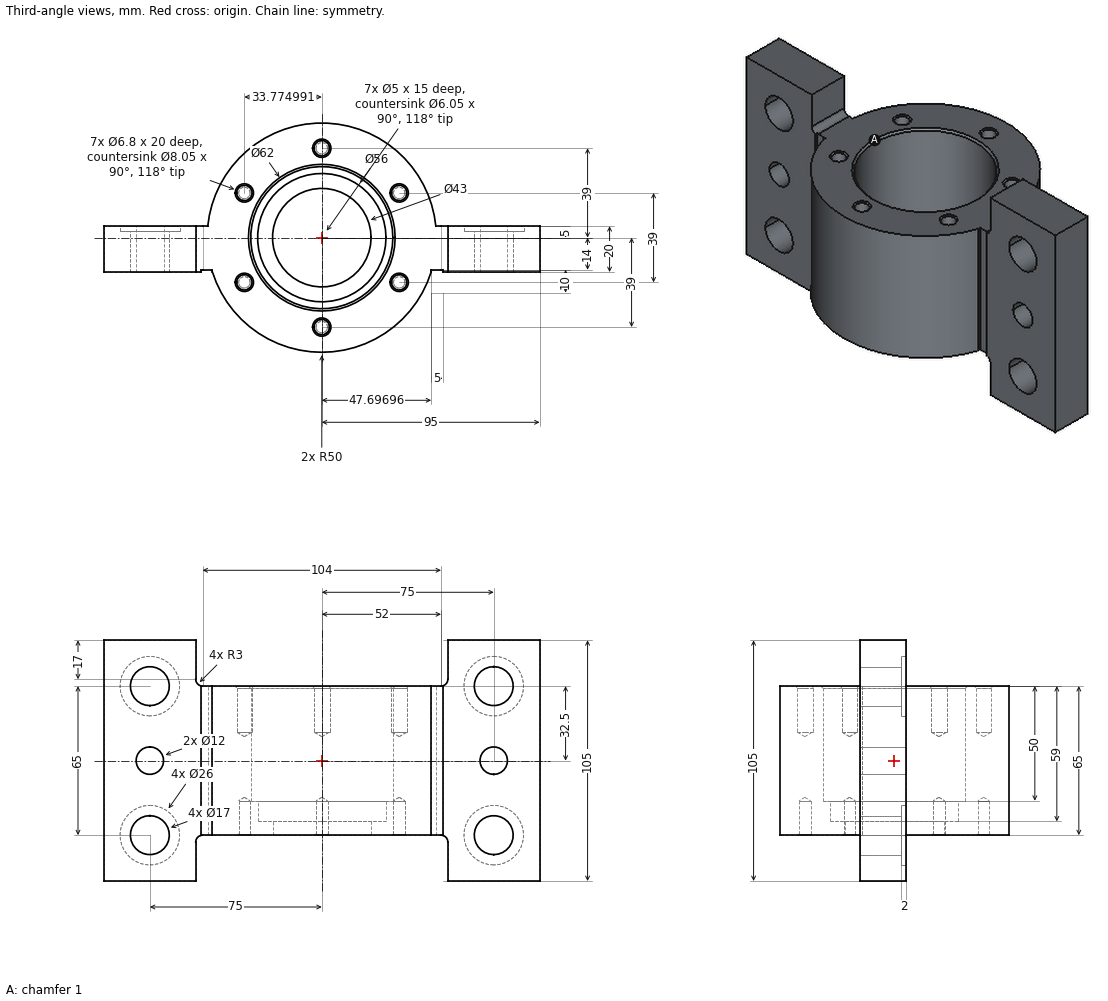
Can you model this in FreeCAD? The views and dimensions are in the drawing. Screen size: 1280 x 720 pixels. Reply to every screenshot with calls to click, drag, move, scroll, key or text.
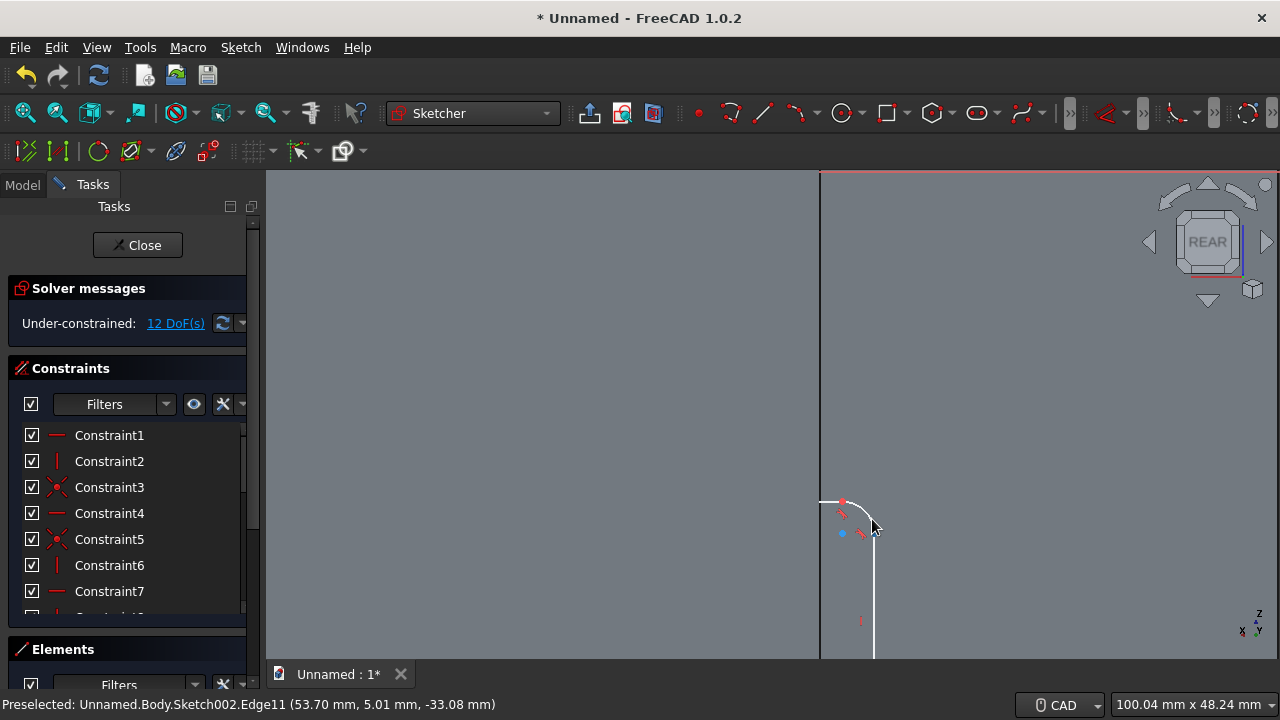
click(871, 519)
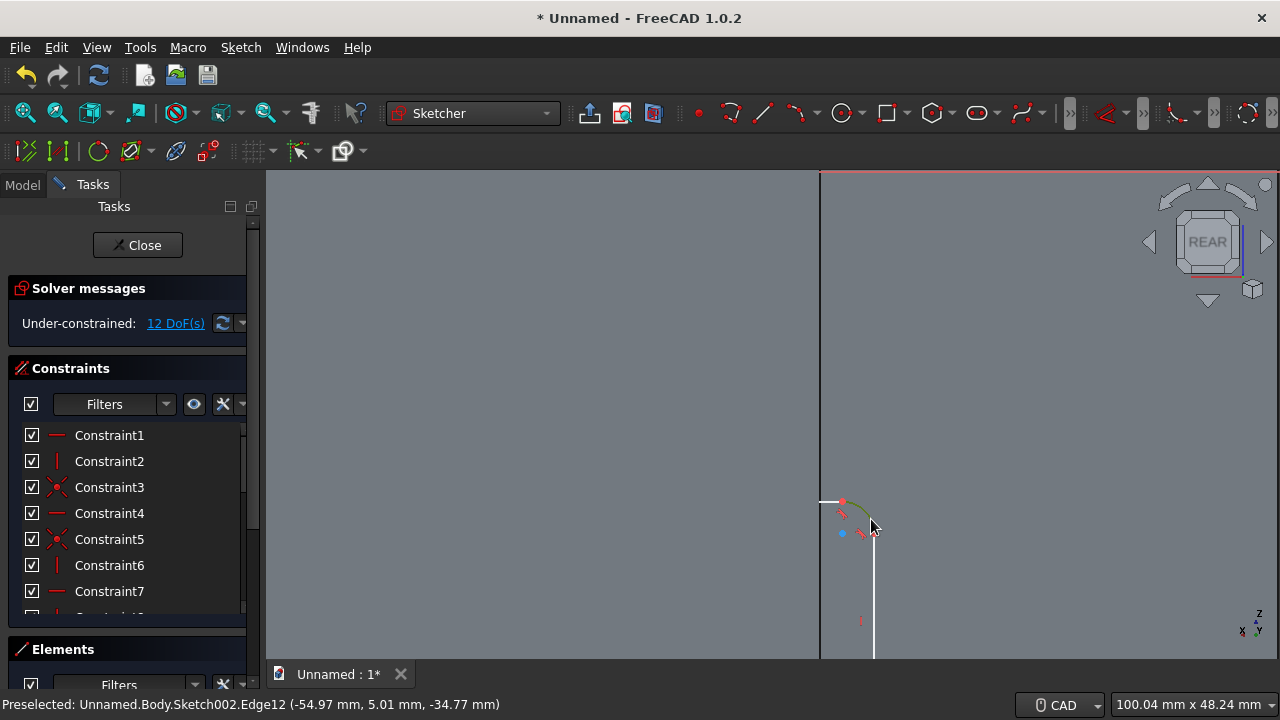
key(e)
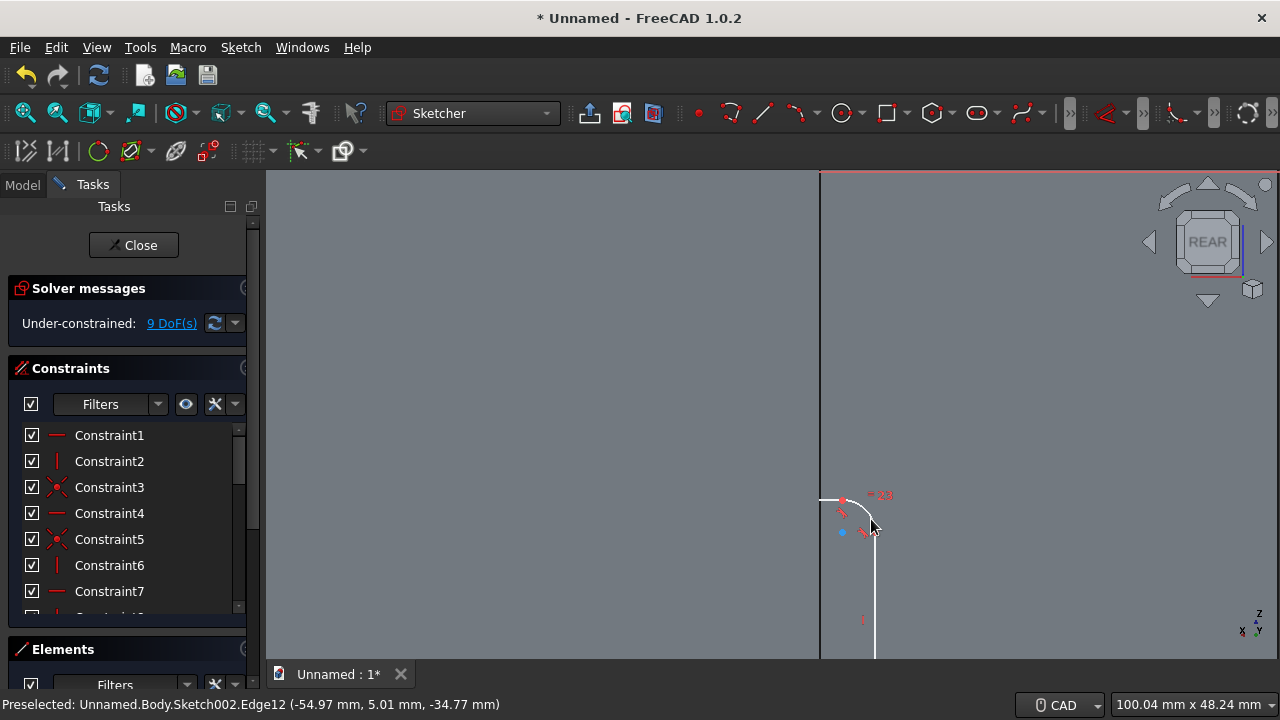
scroll(872, 519, down, 6)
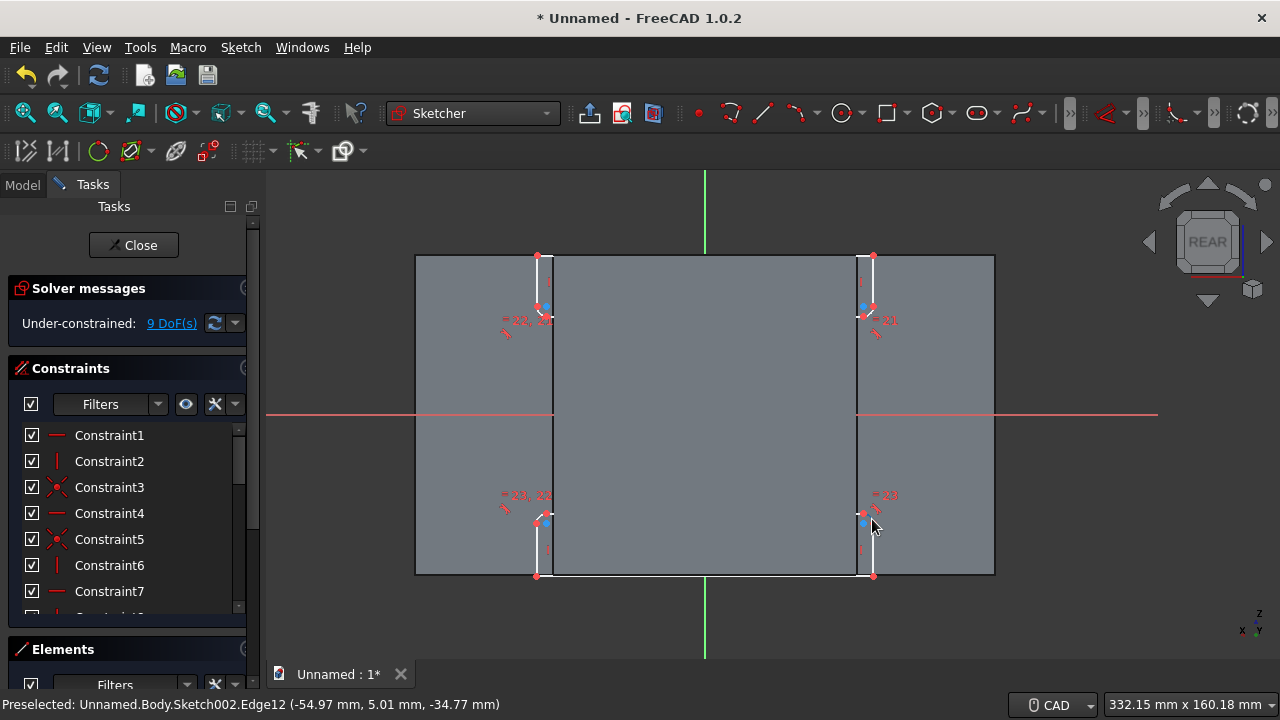
scroll(547, 307, up, 2)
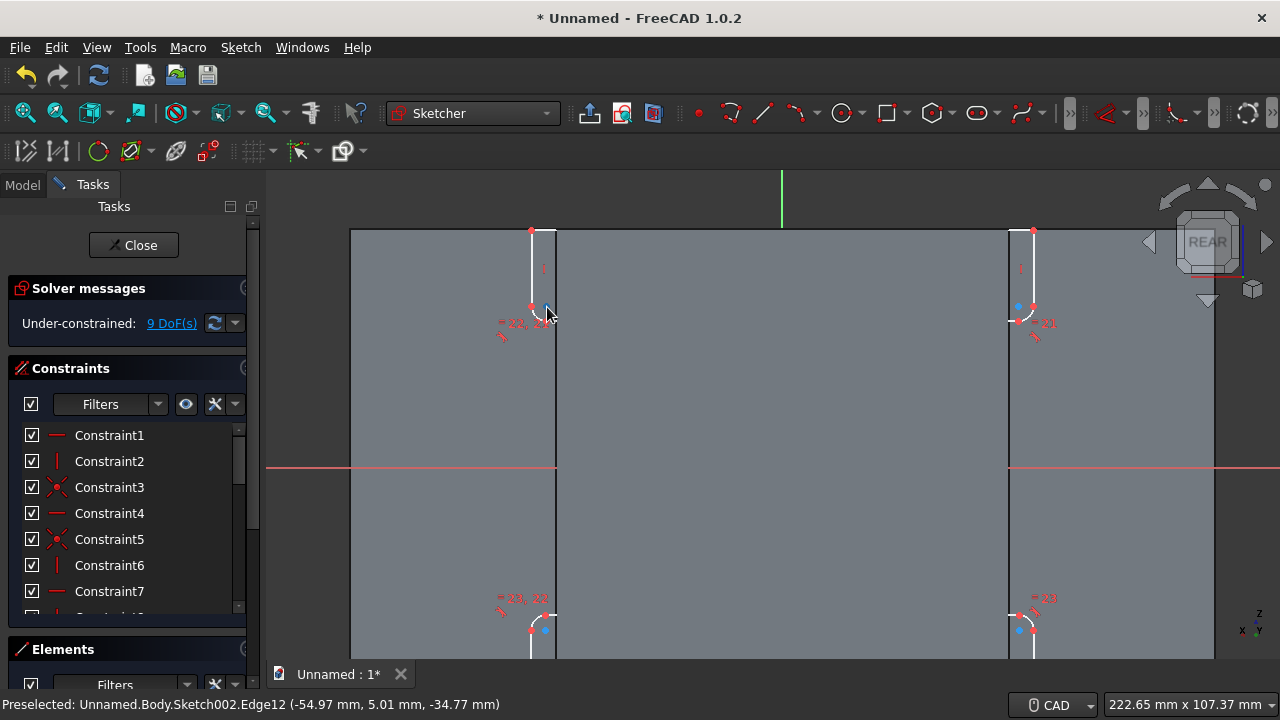
click(547, 306)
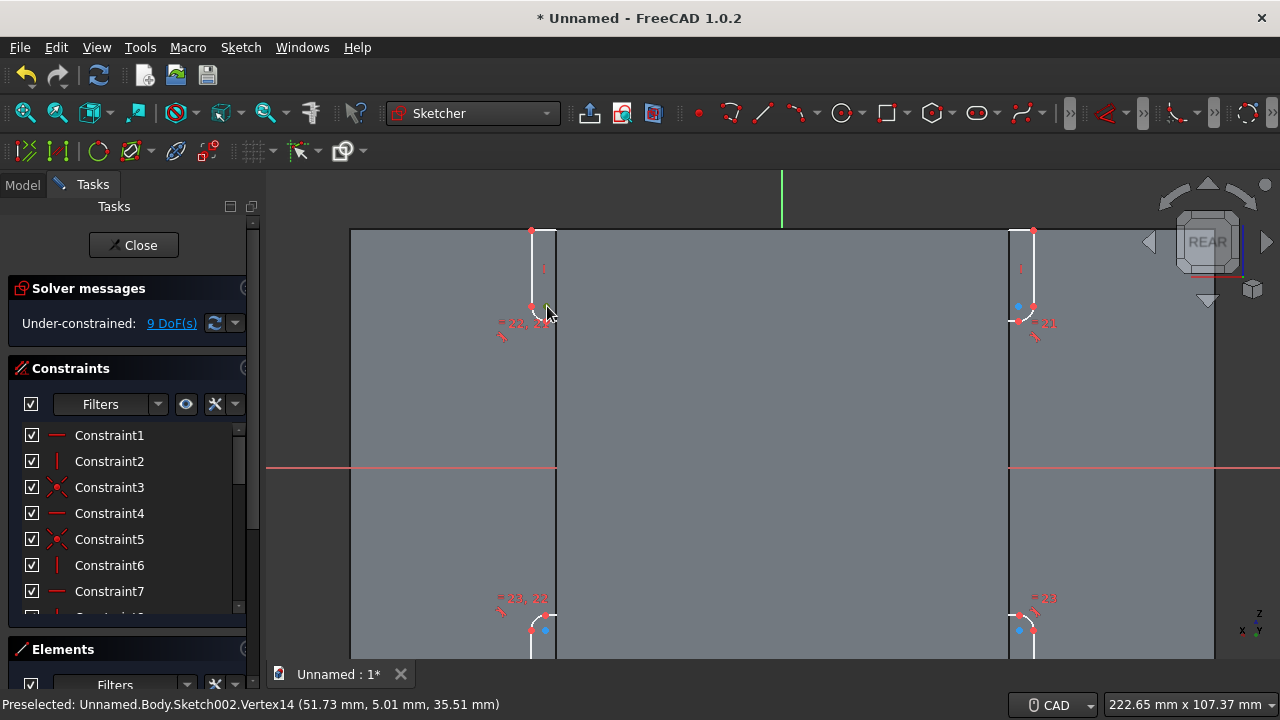
click(546, 630)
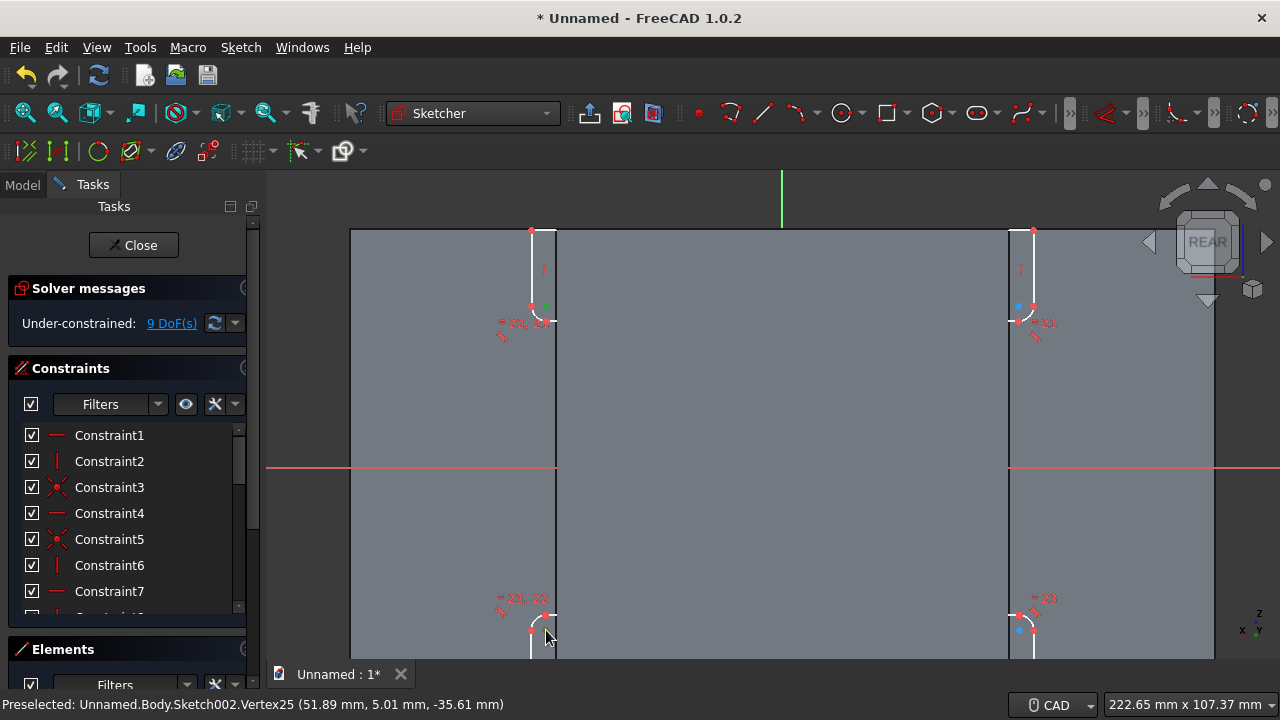
click(353, 468)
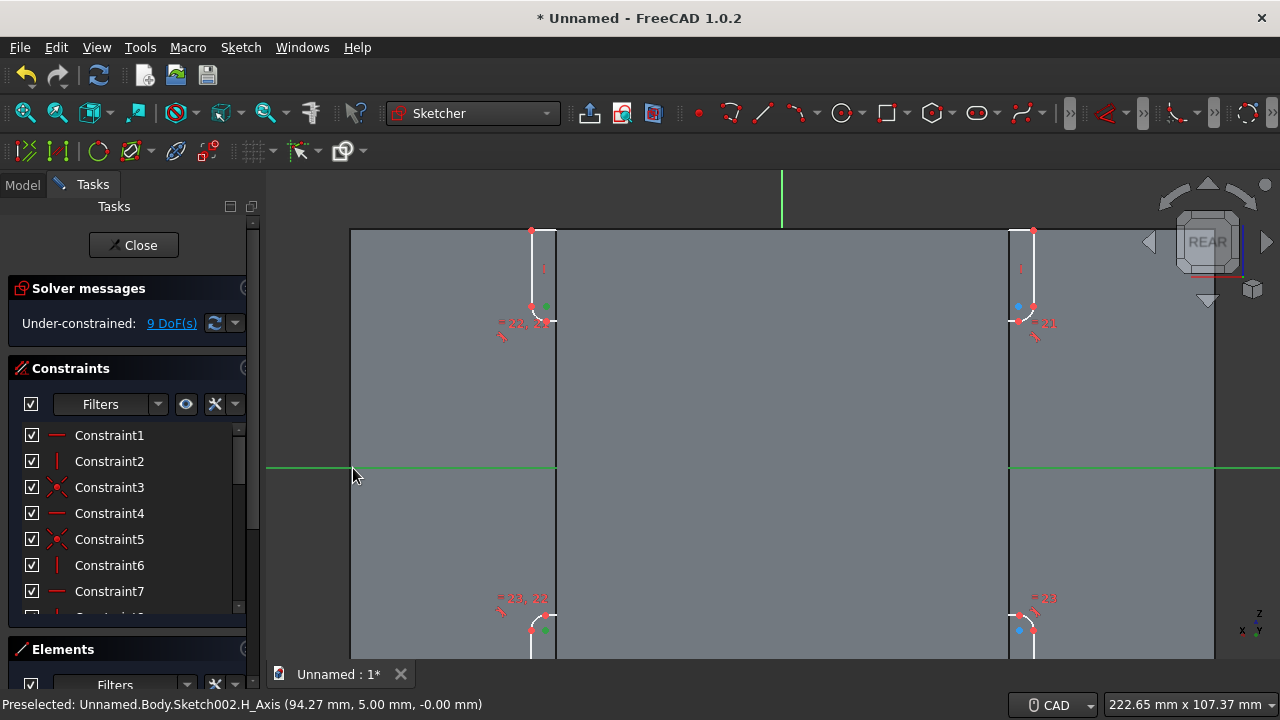
key(s)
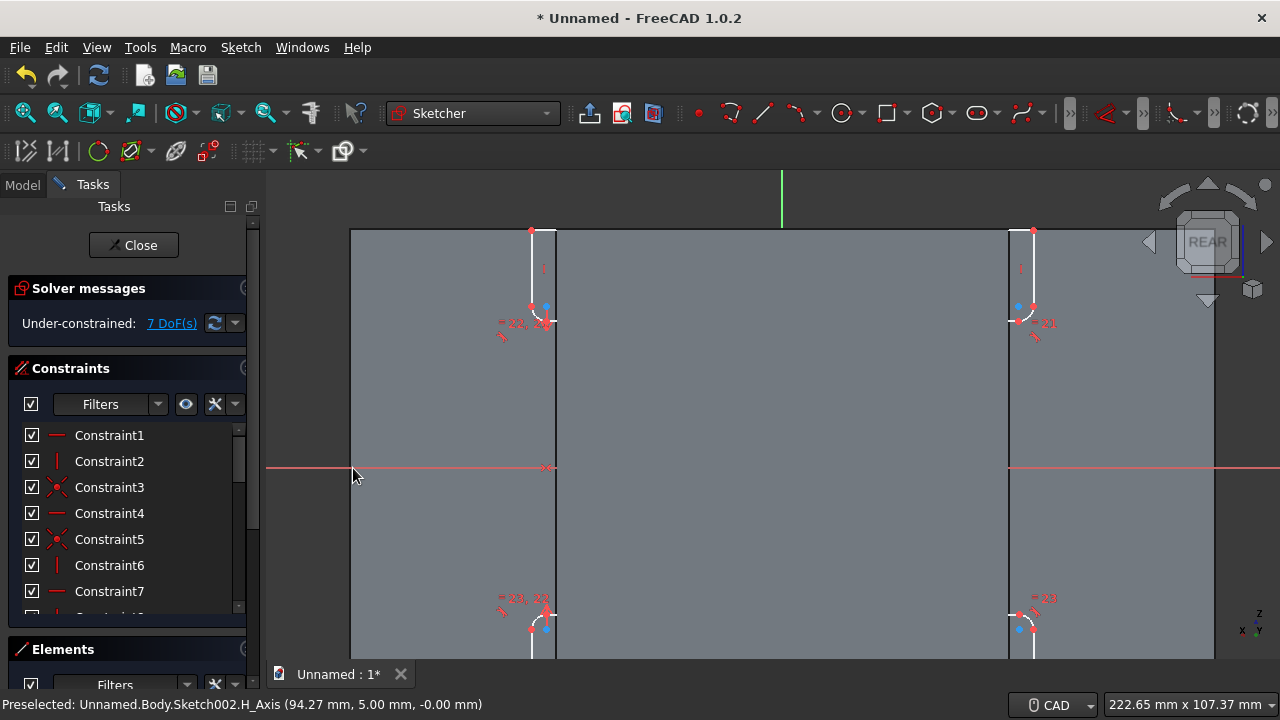
click(1034, 230)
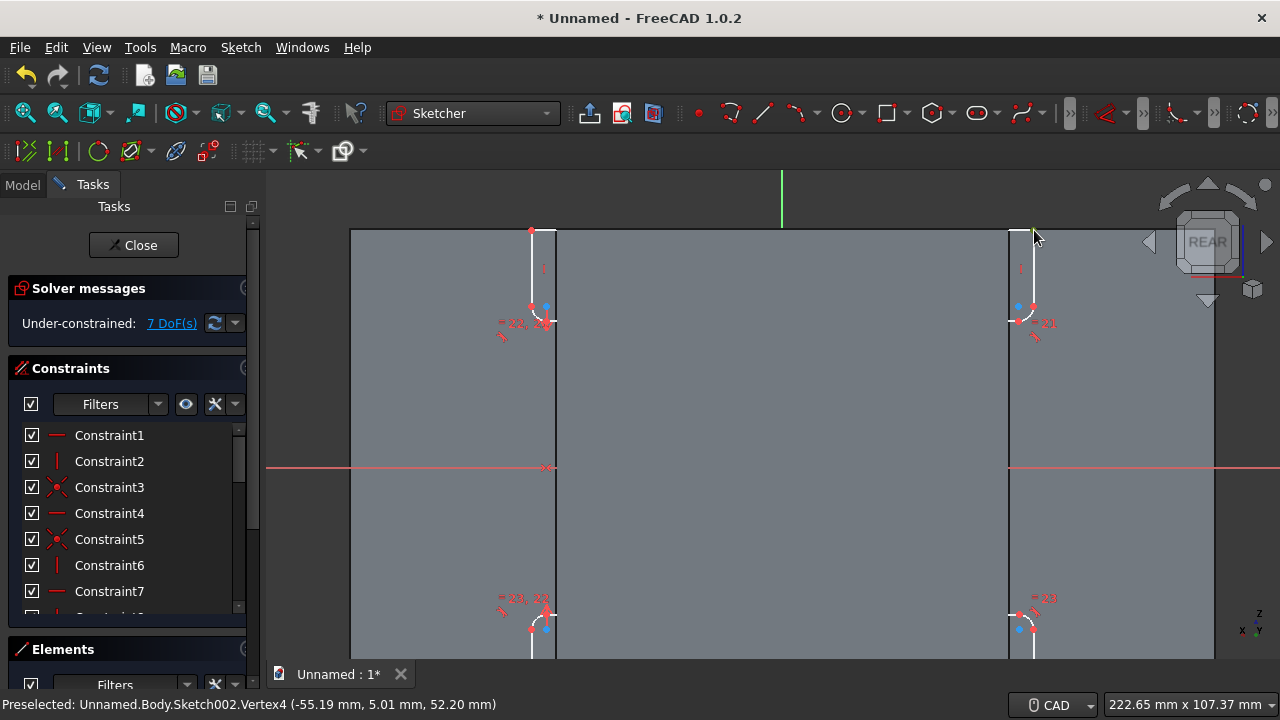
scroll(546, 306, down, 2)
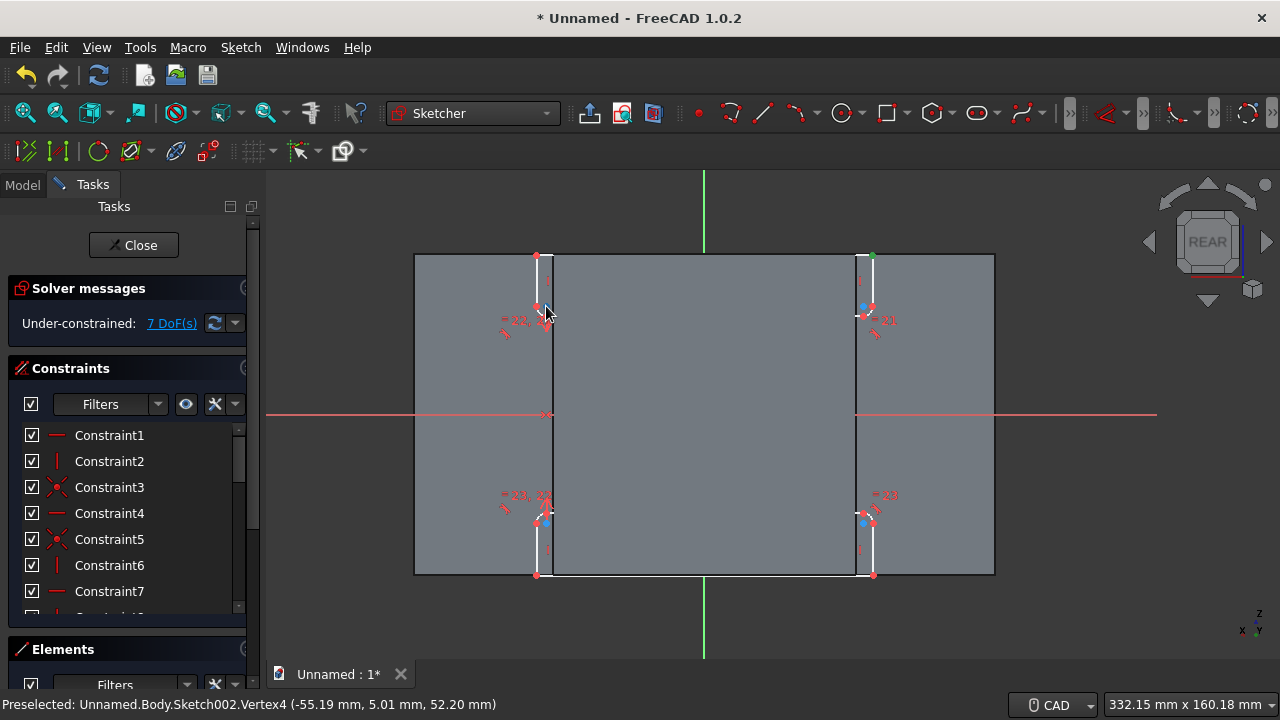
click(873, 576)